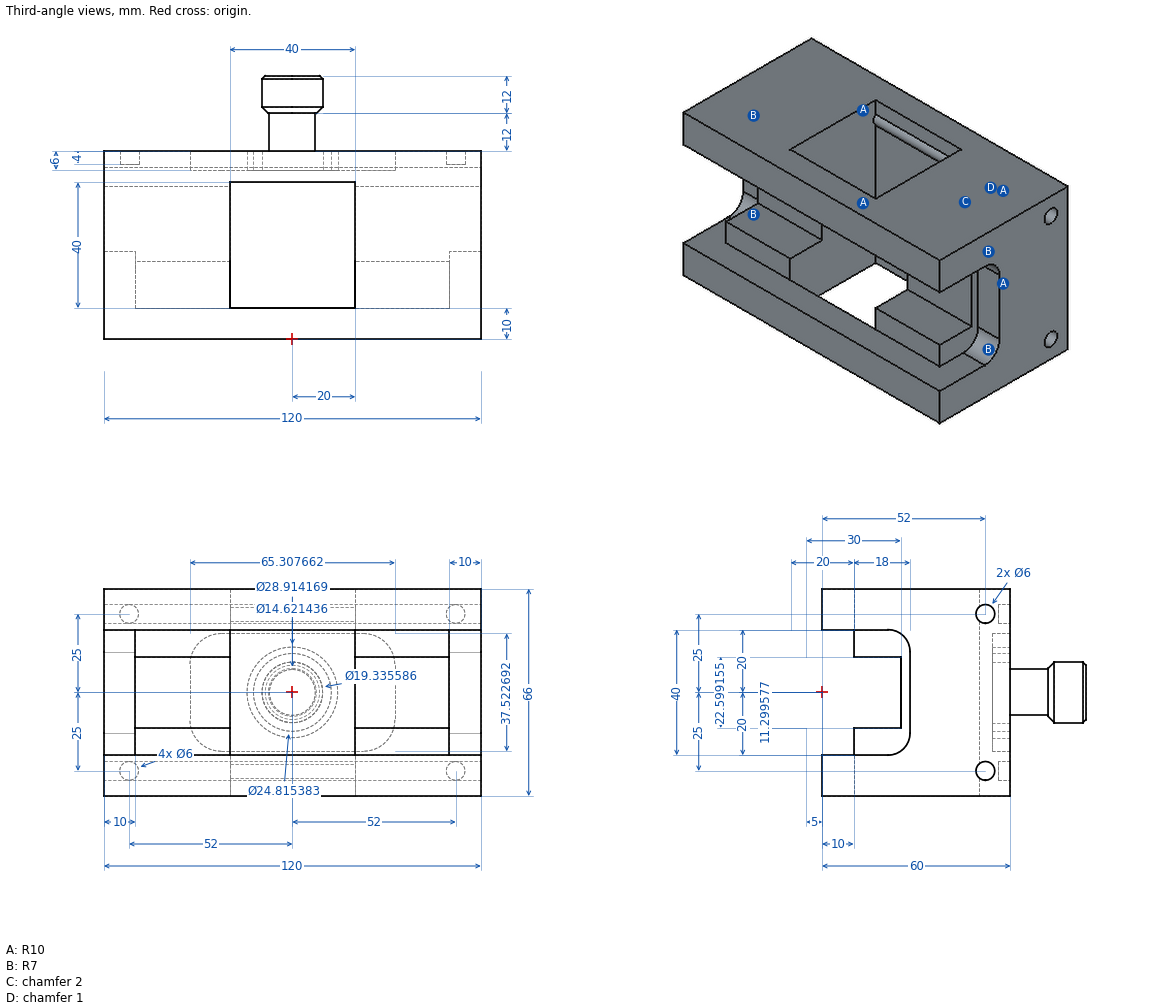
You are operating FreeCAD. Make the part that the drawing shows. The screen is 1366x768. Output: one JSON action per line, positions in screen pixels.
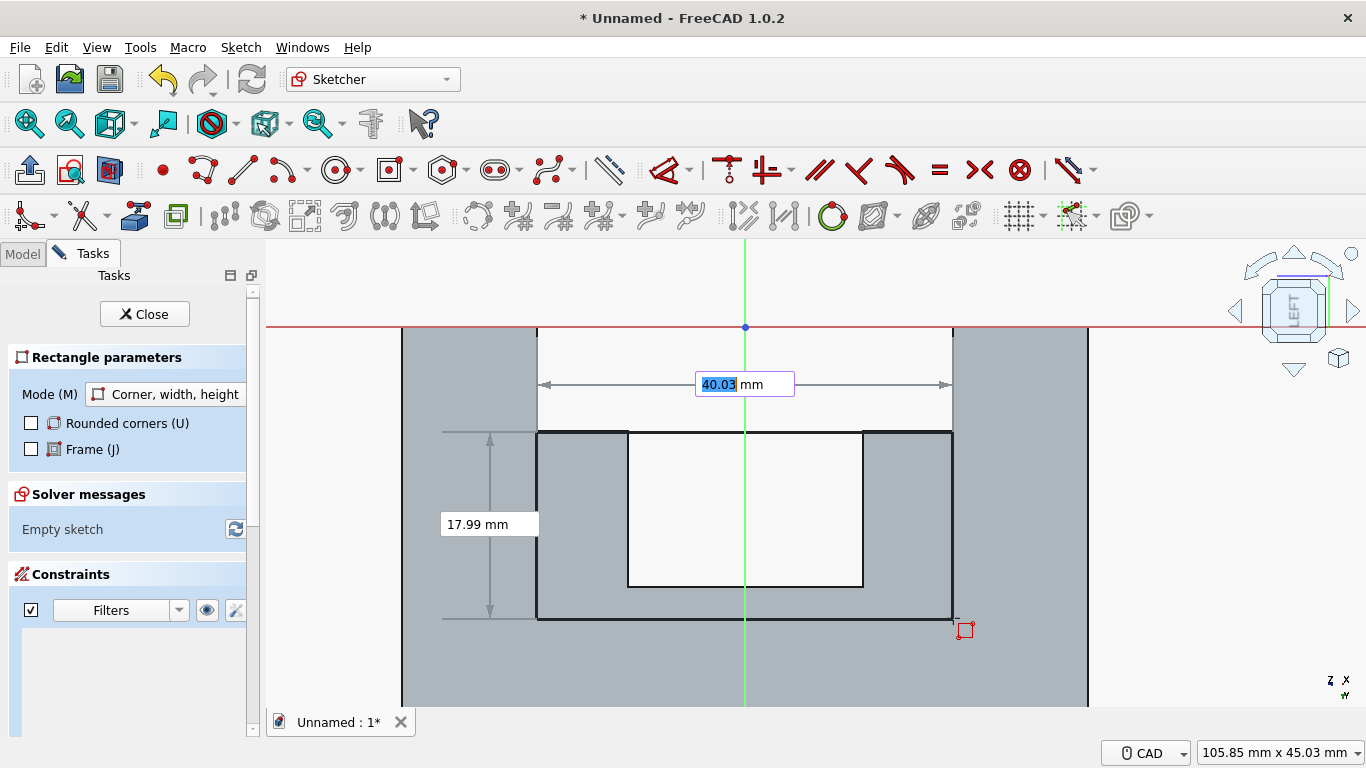
{"action": "type", "text": "40"}
{"action": "key", "text": "Tab"}
{"action": "type", "text": "18"}
{"action": "key", "text": "Return"}
{"action": "key", "text": "Escape"}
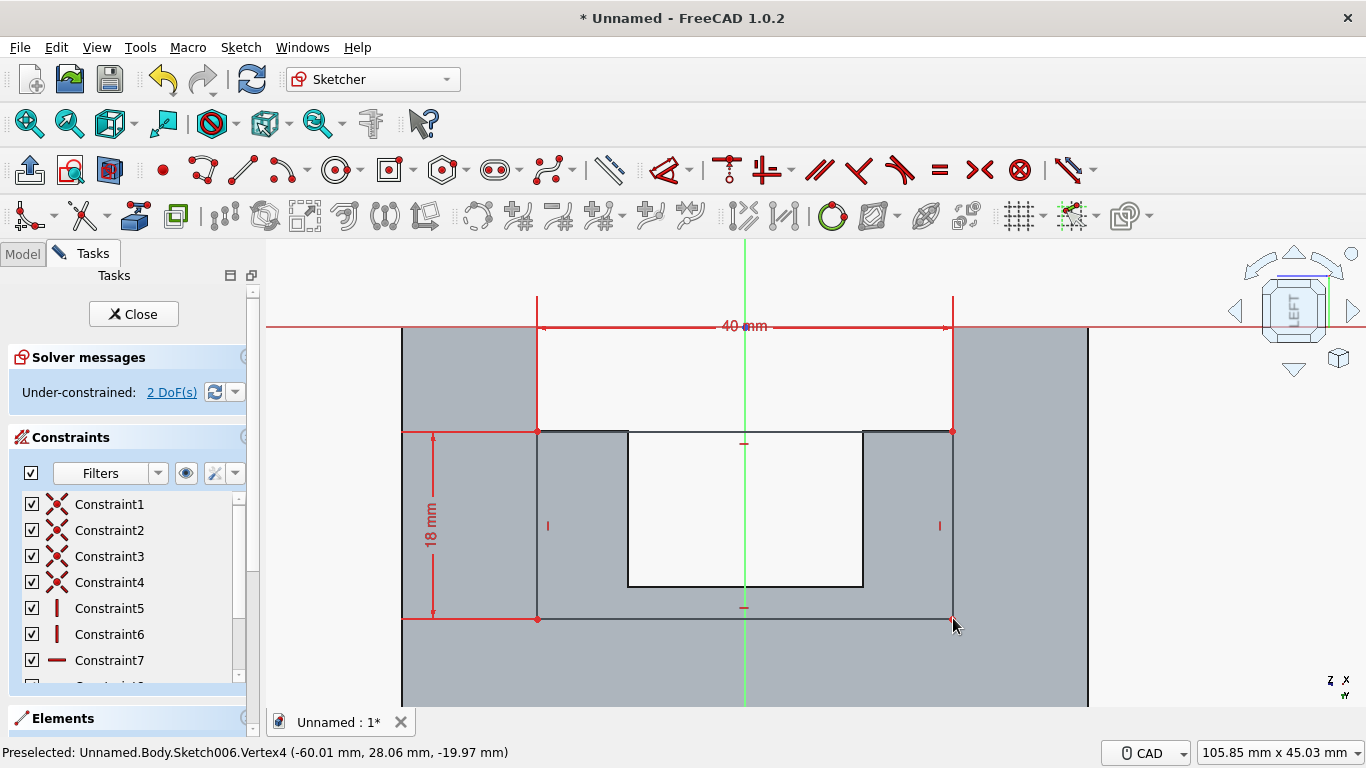
{"action": "left_click", "coordinate": [664, 170]}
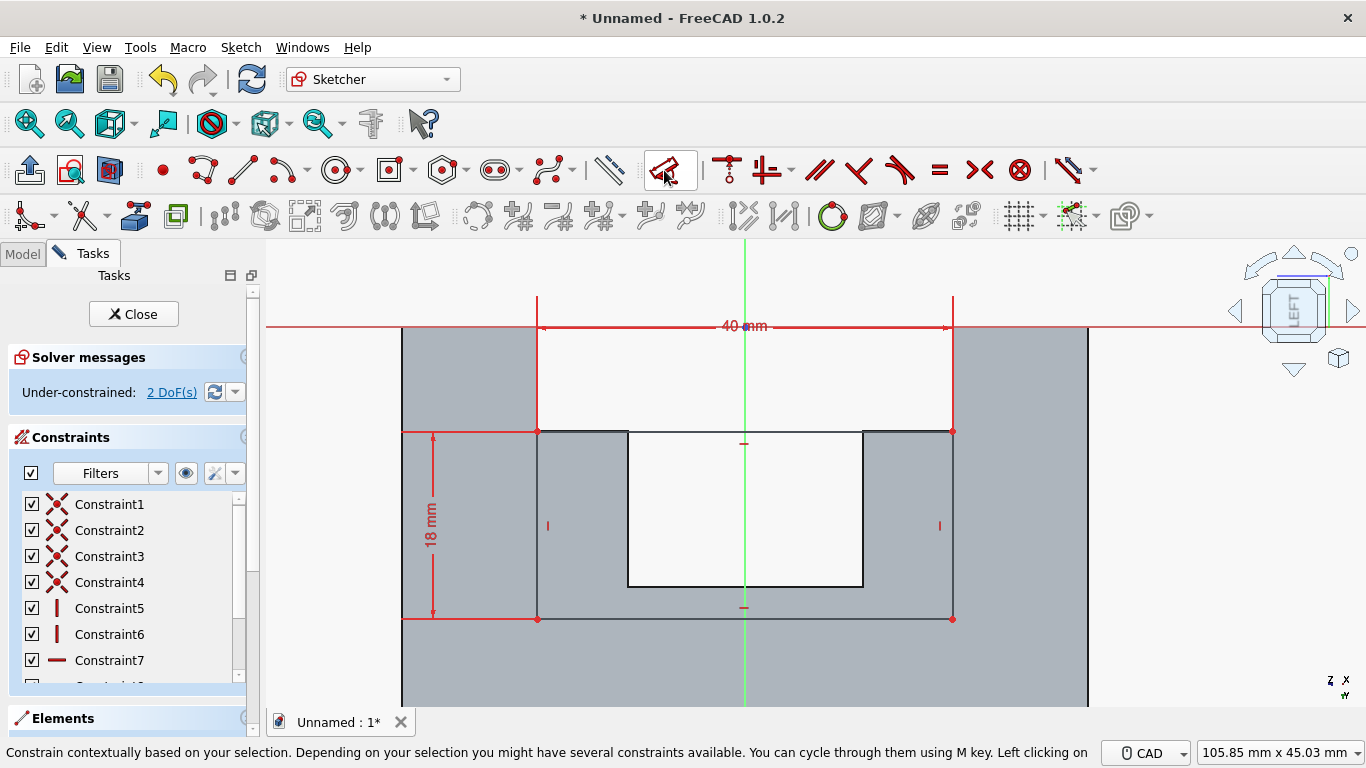
{"action": "left_click", "coordinate": [537, 432]}
{"action": "left_click", "coordinate": [641, 293]}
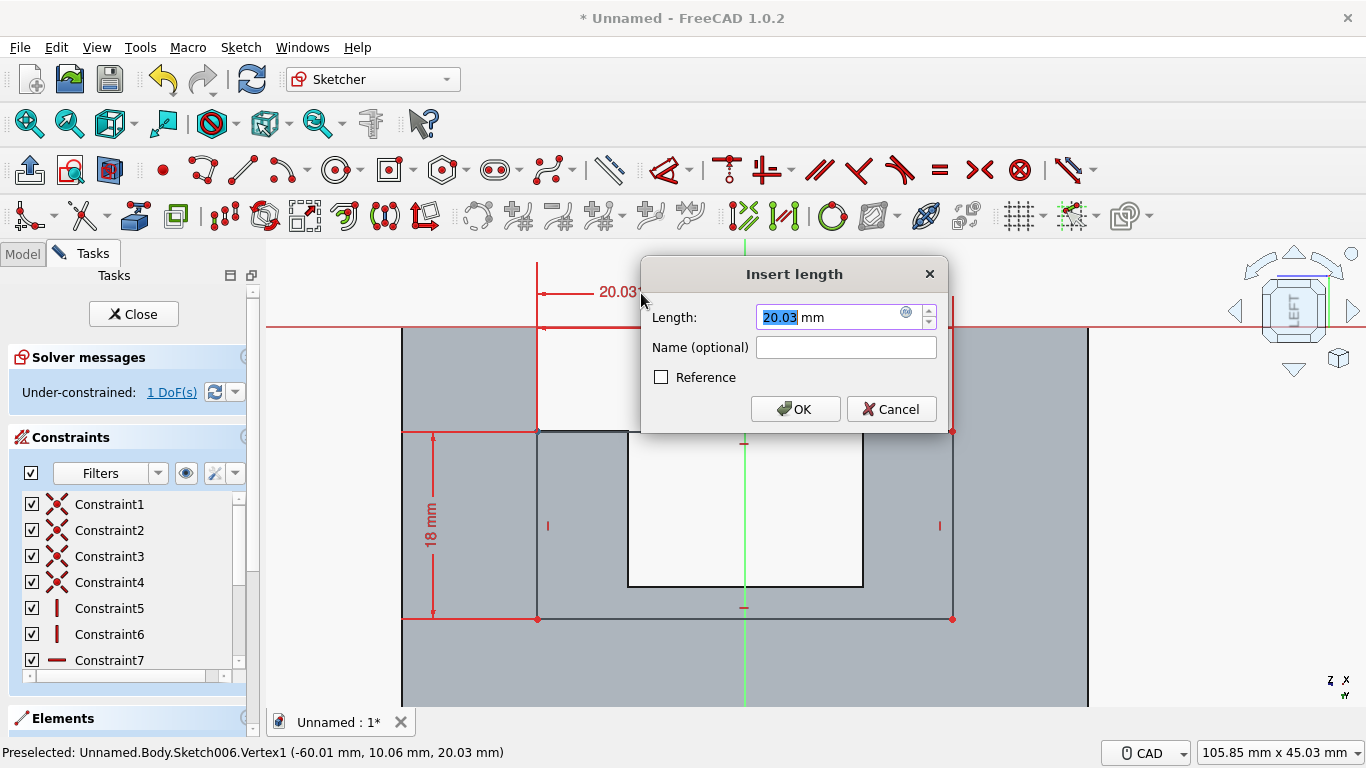
{"action": "type", "text": "20"}
{"action": "key", "text": "Return"}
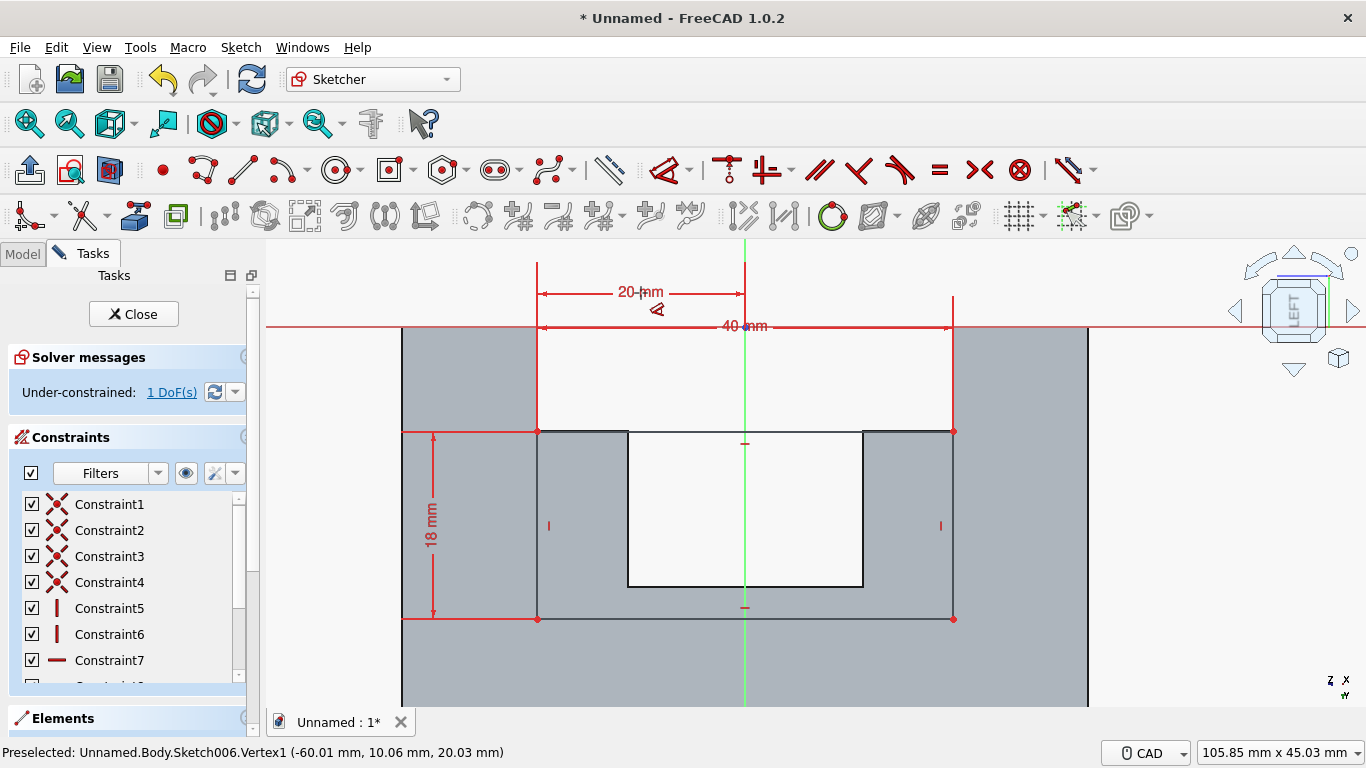
{"action": "left_click", "coordinate": [537, 432]}
{"action": "left_click", "coordinate": [503, 380]}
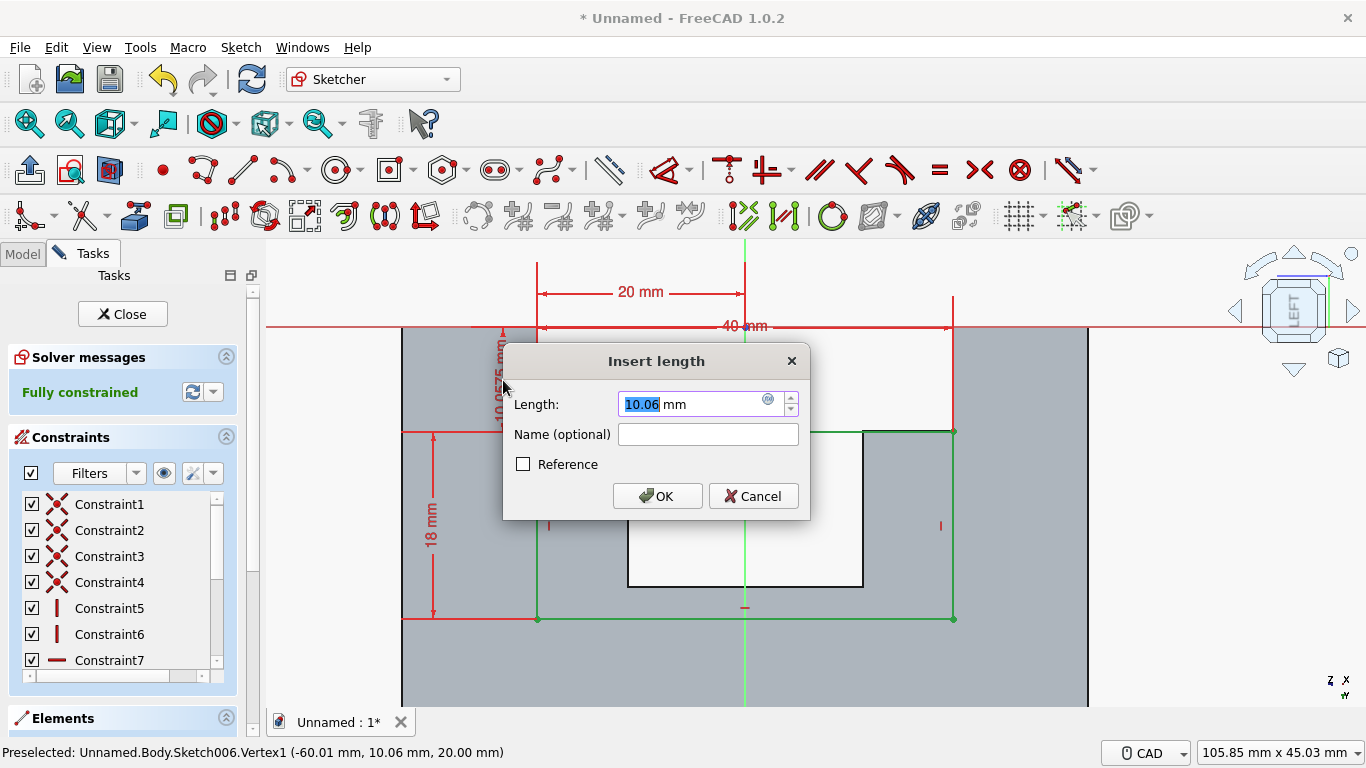
{"action": "type", "text": "10"}
{"action": "key", "text": "Return"}
{"action": "key", "text": "Escape"}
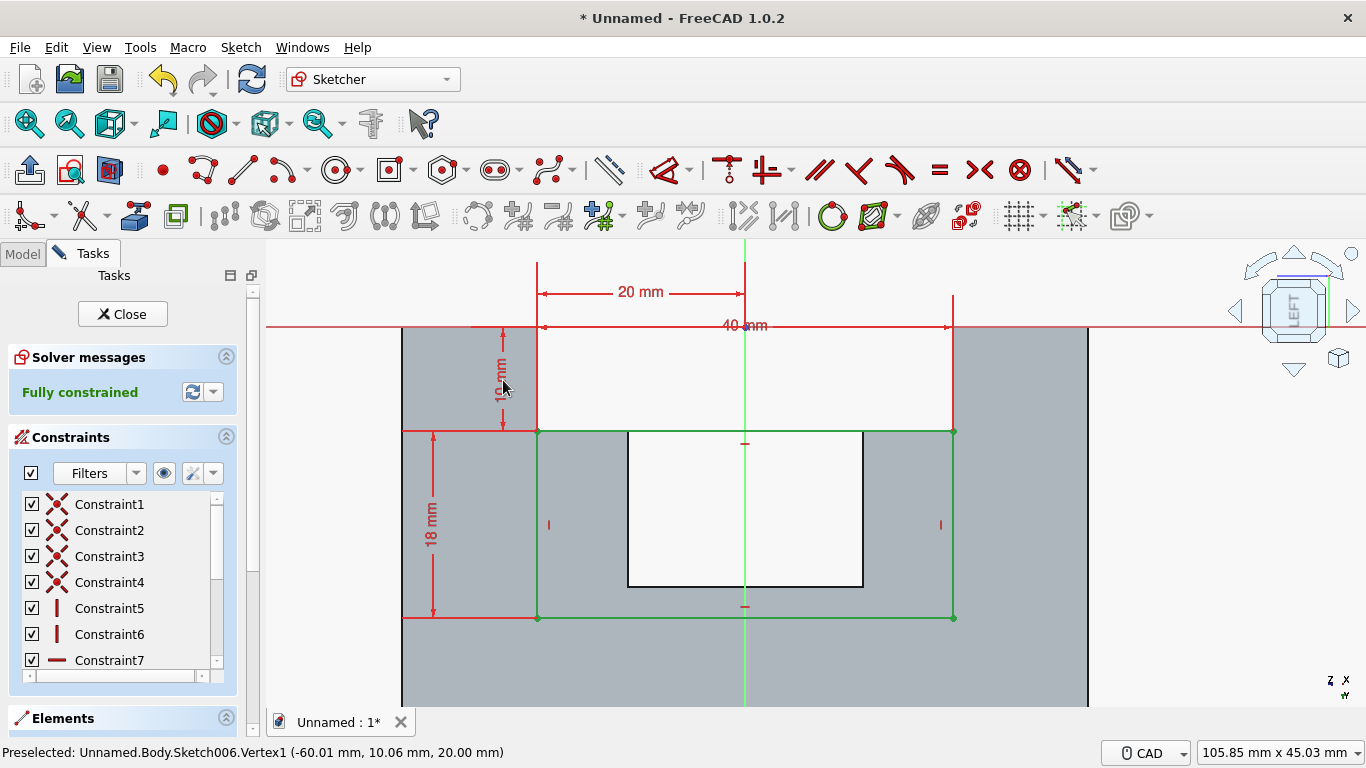
{"action": "left_click", "coordinate": [123, 314]}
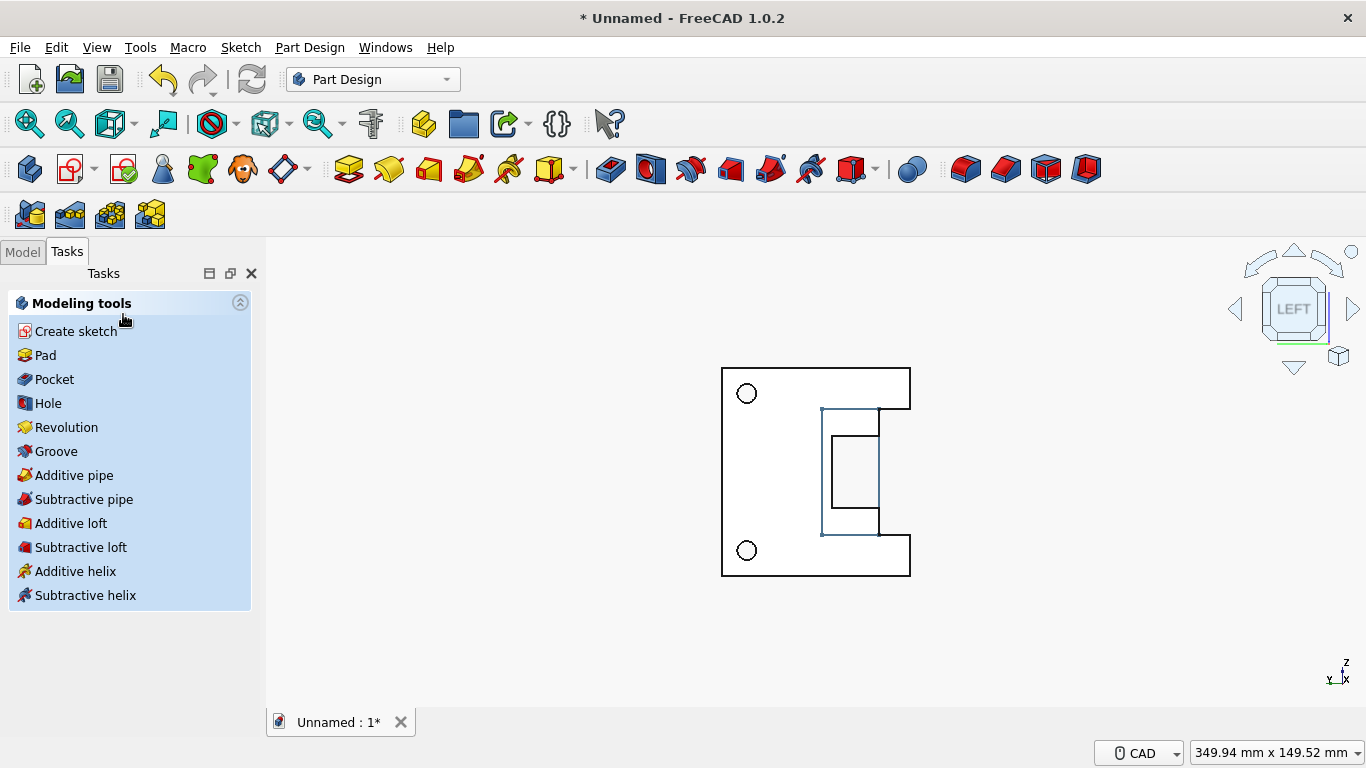
{"action": "left_click", "coordinate": [612, 170]}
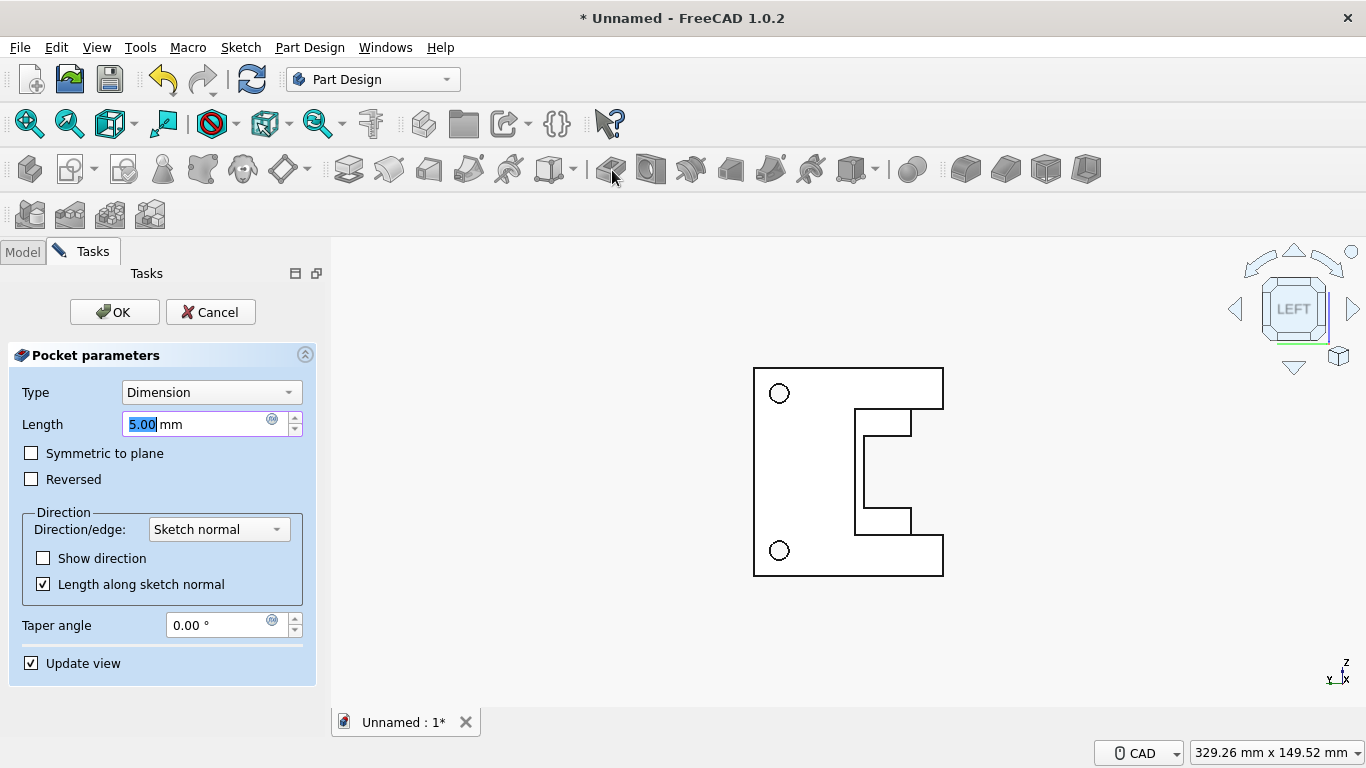
{"action": "type", "text": "10"}
{"action": "key", "text": "Tab"}